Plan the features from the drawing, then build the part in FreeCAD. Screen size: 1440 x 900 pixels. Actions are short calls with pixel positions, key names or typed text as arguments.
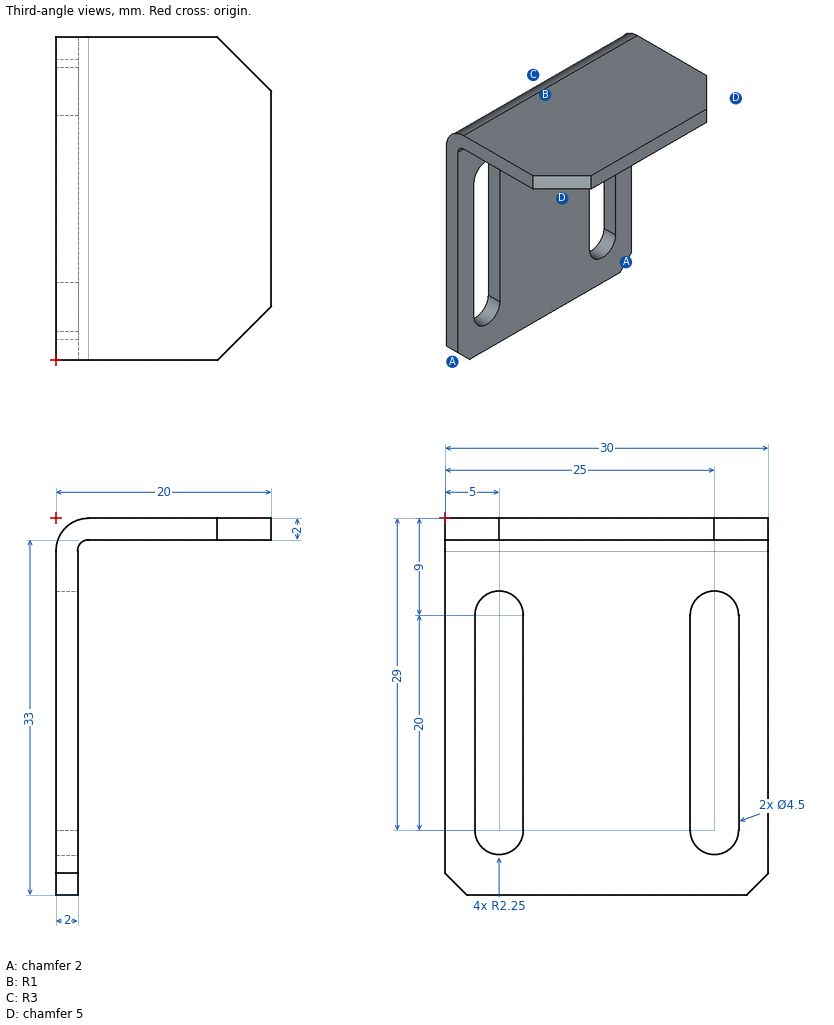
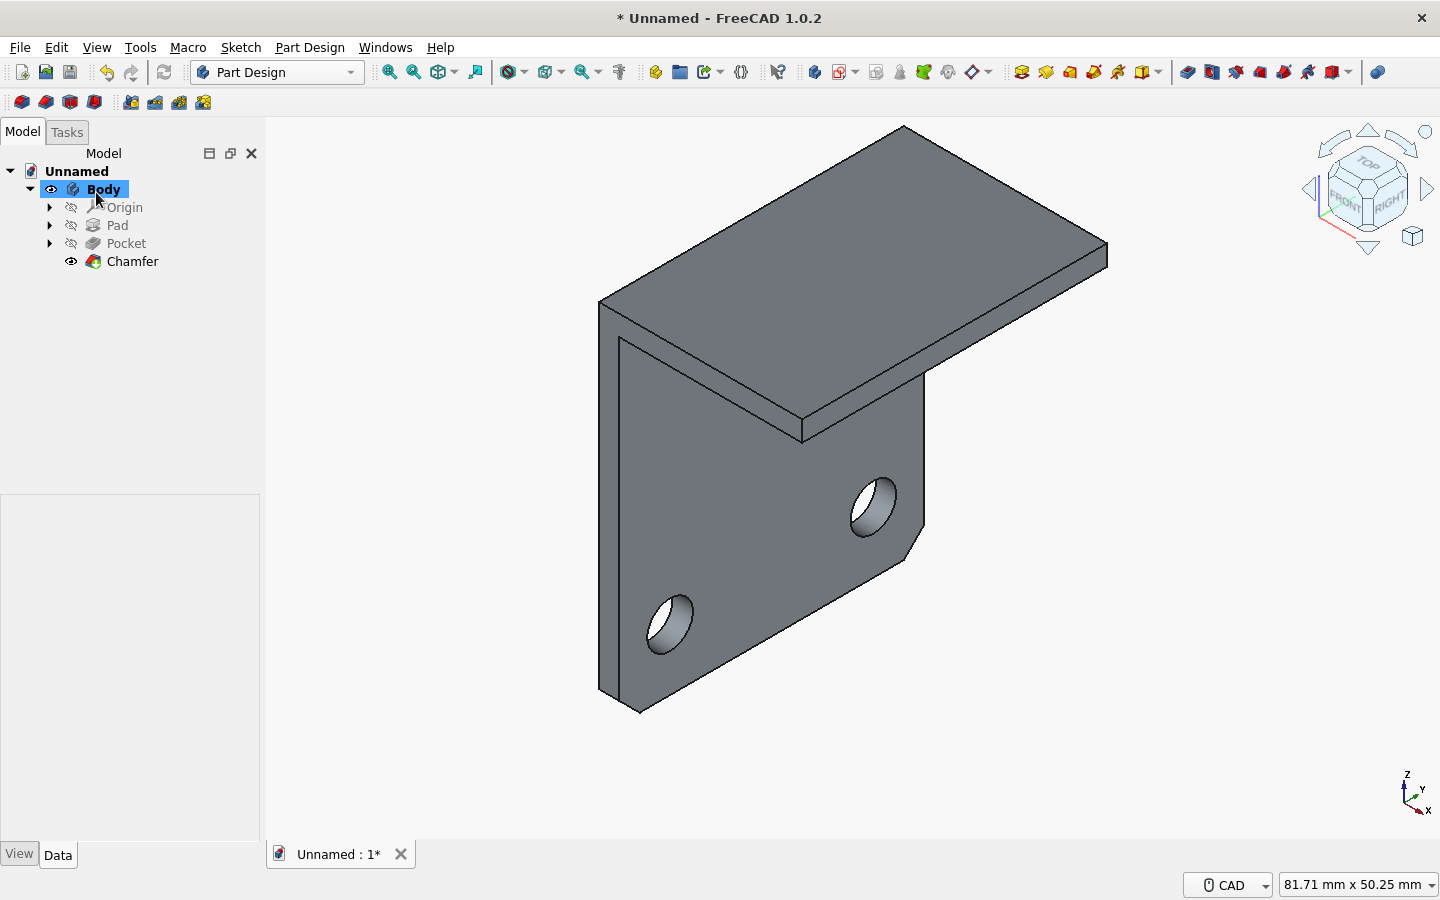
key(2)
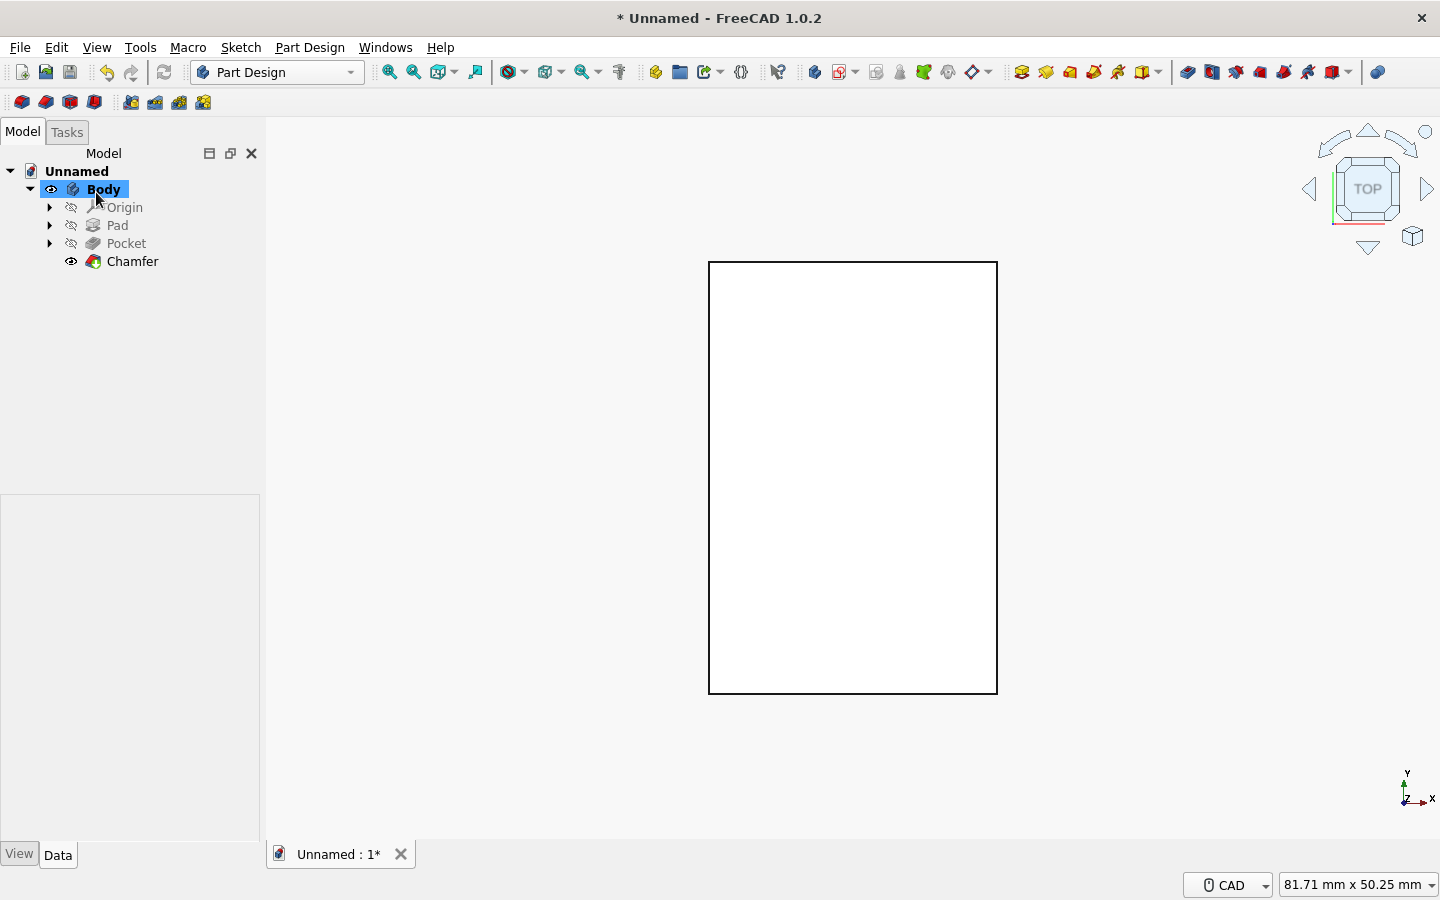
key(1)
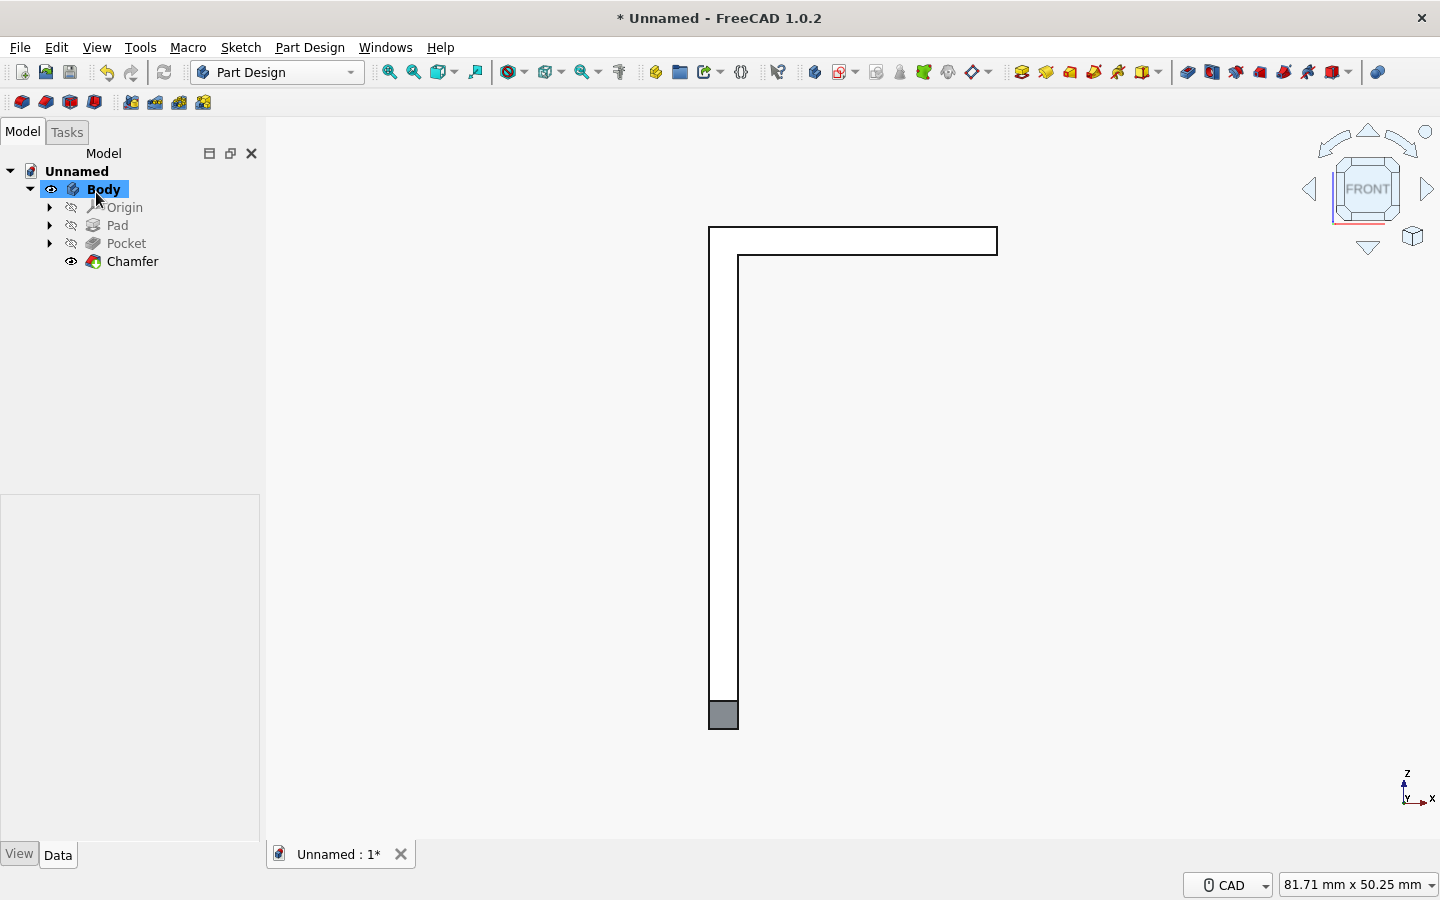
key(3)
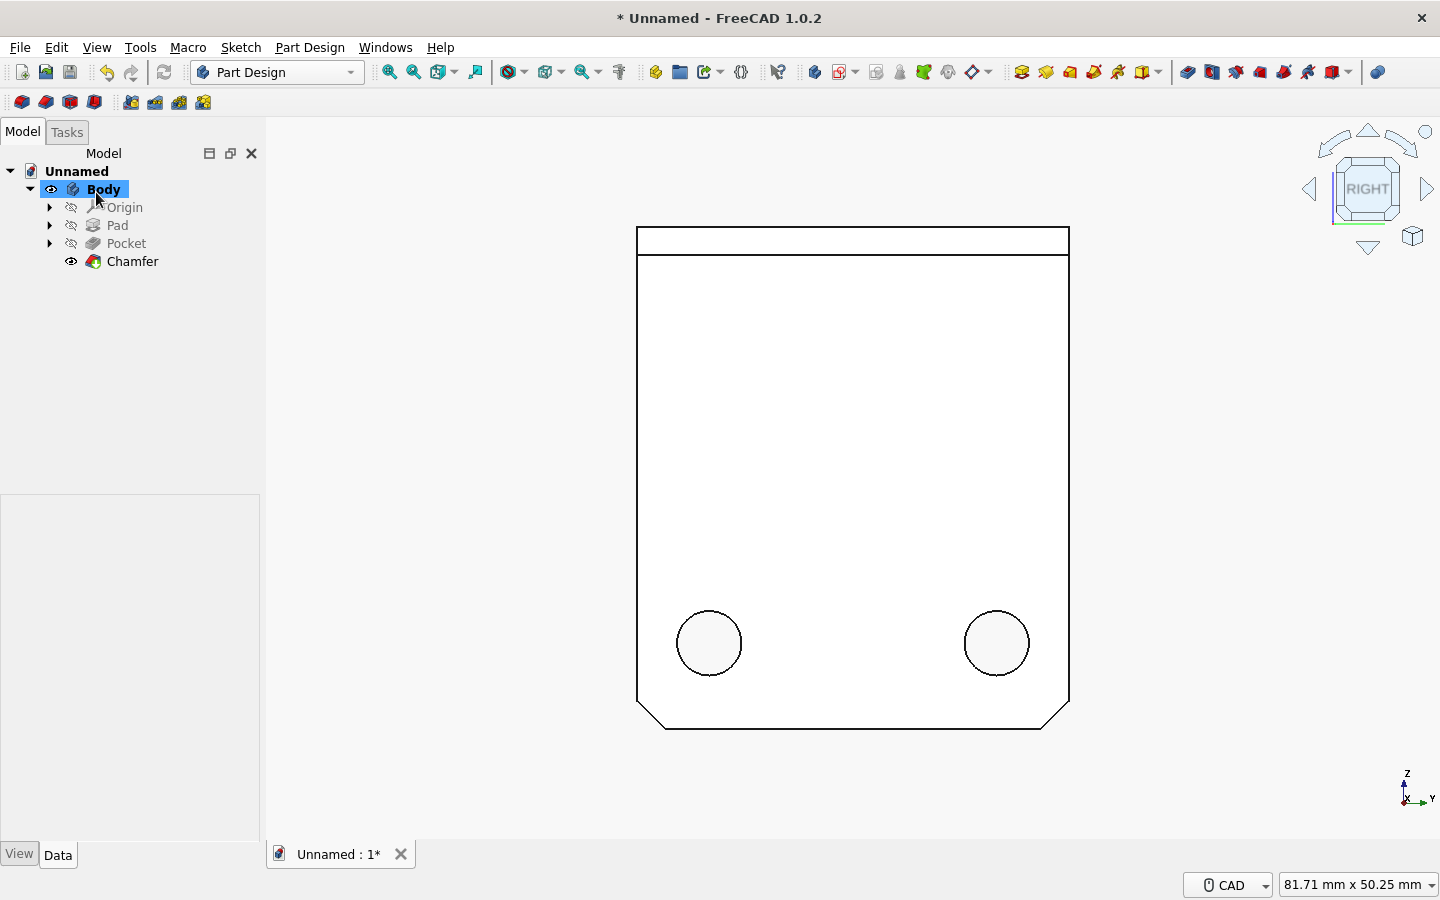
key(5)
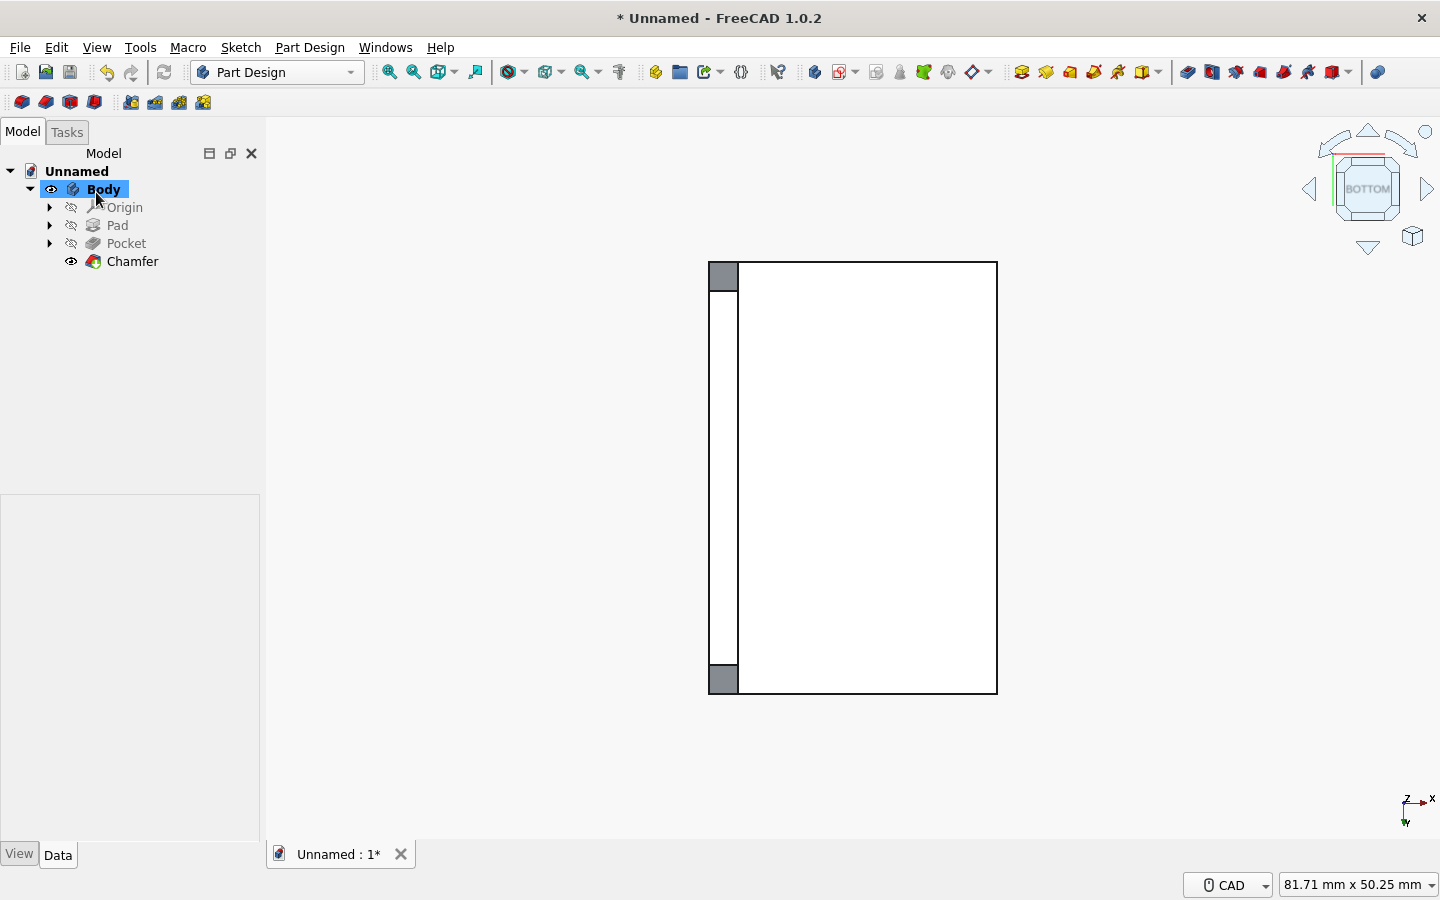
key(4)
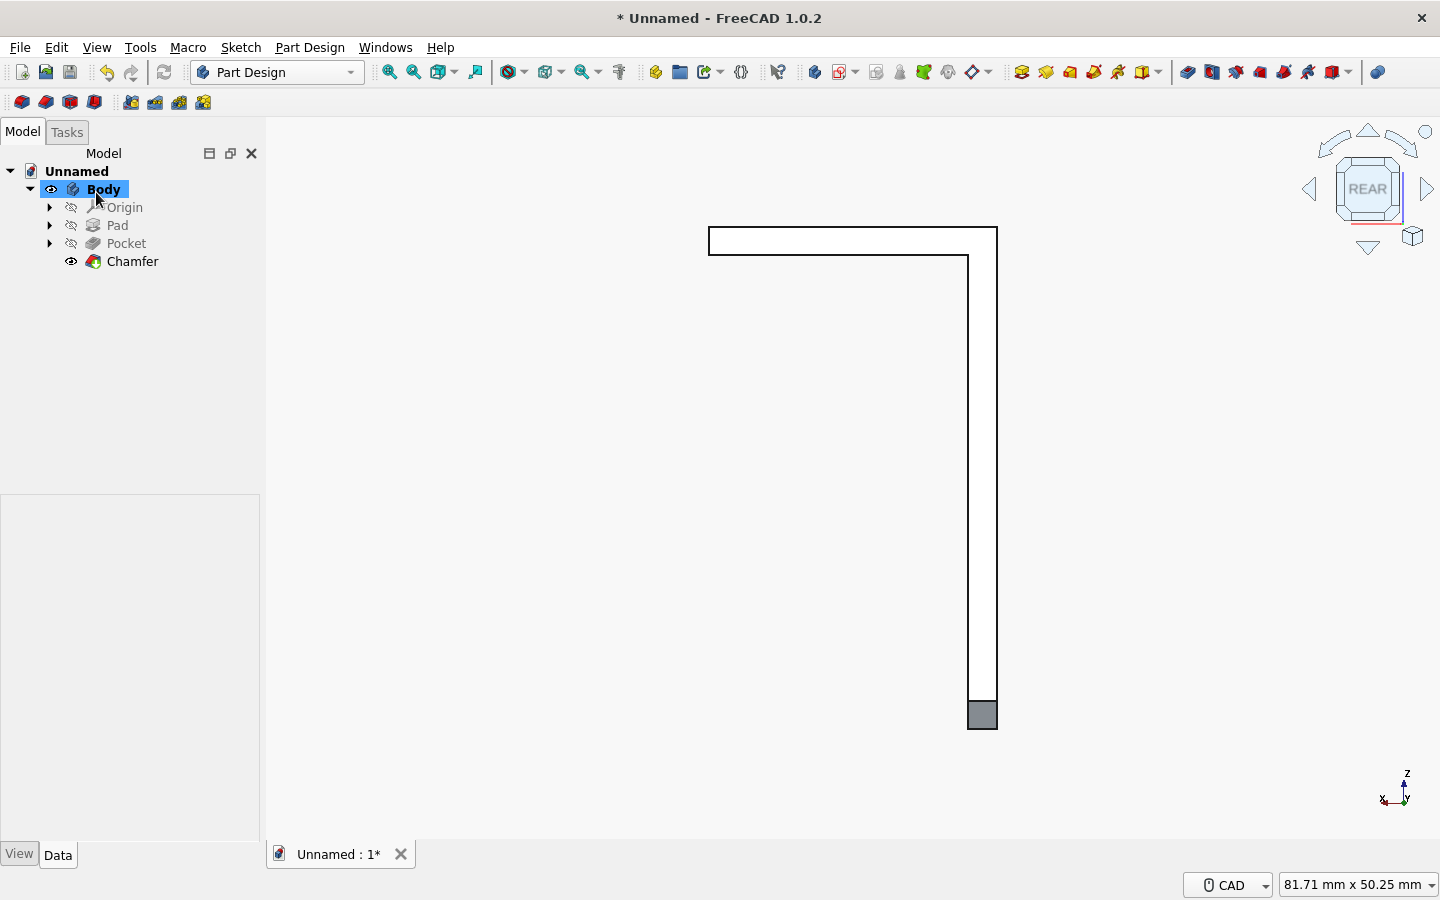
key(6)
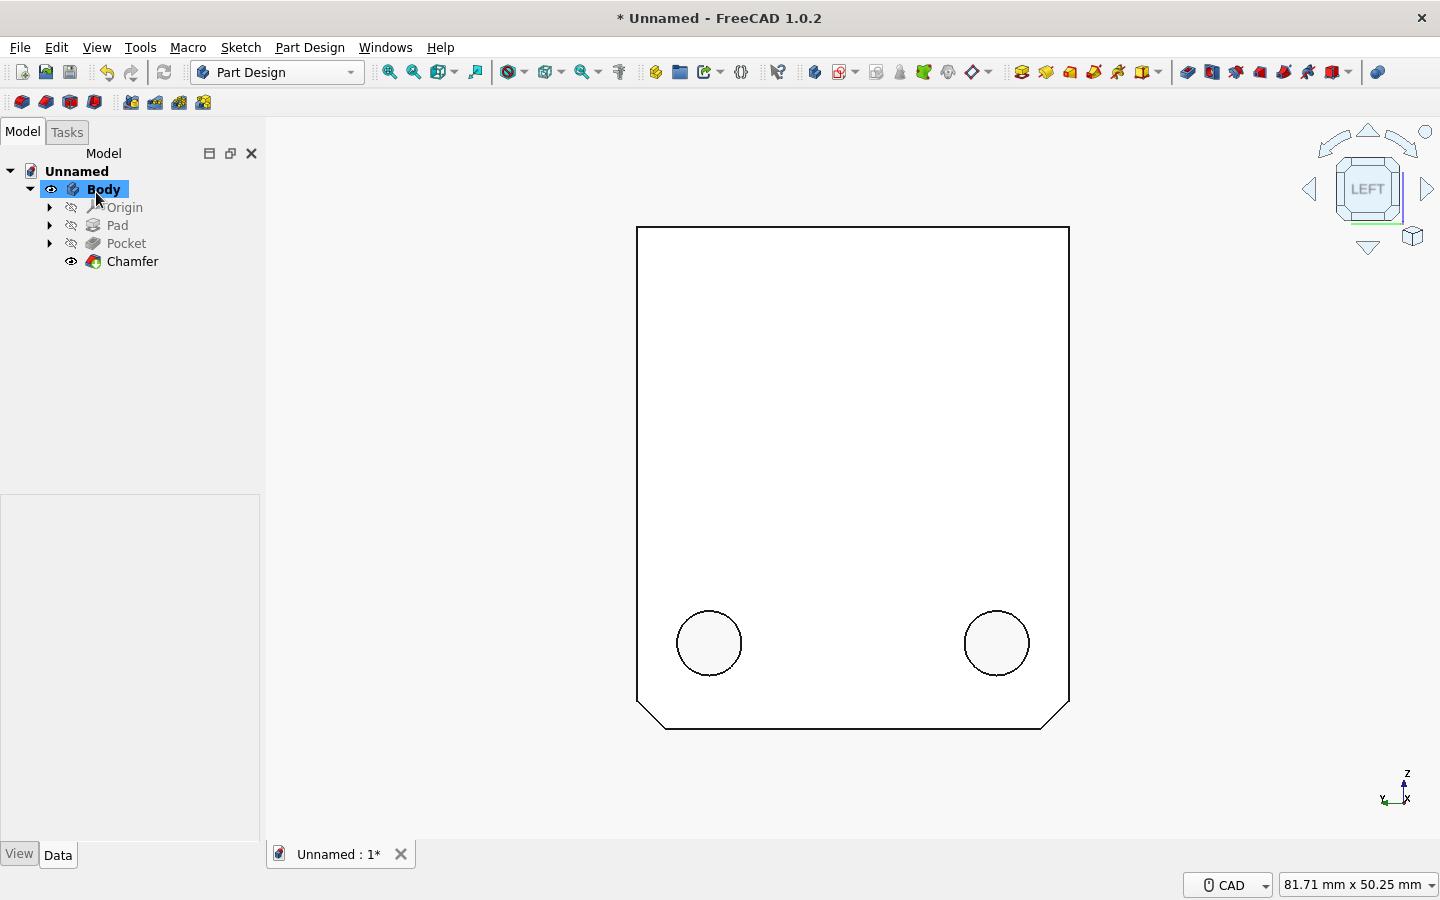
key(v)
key(3)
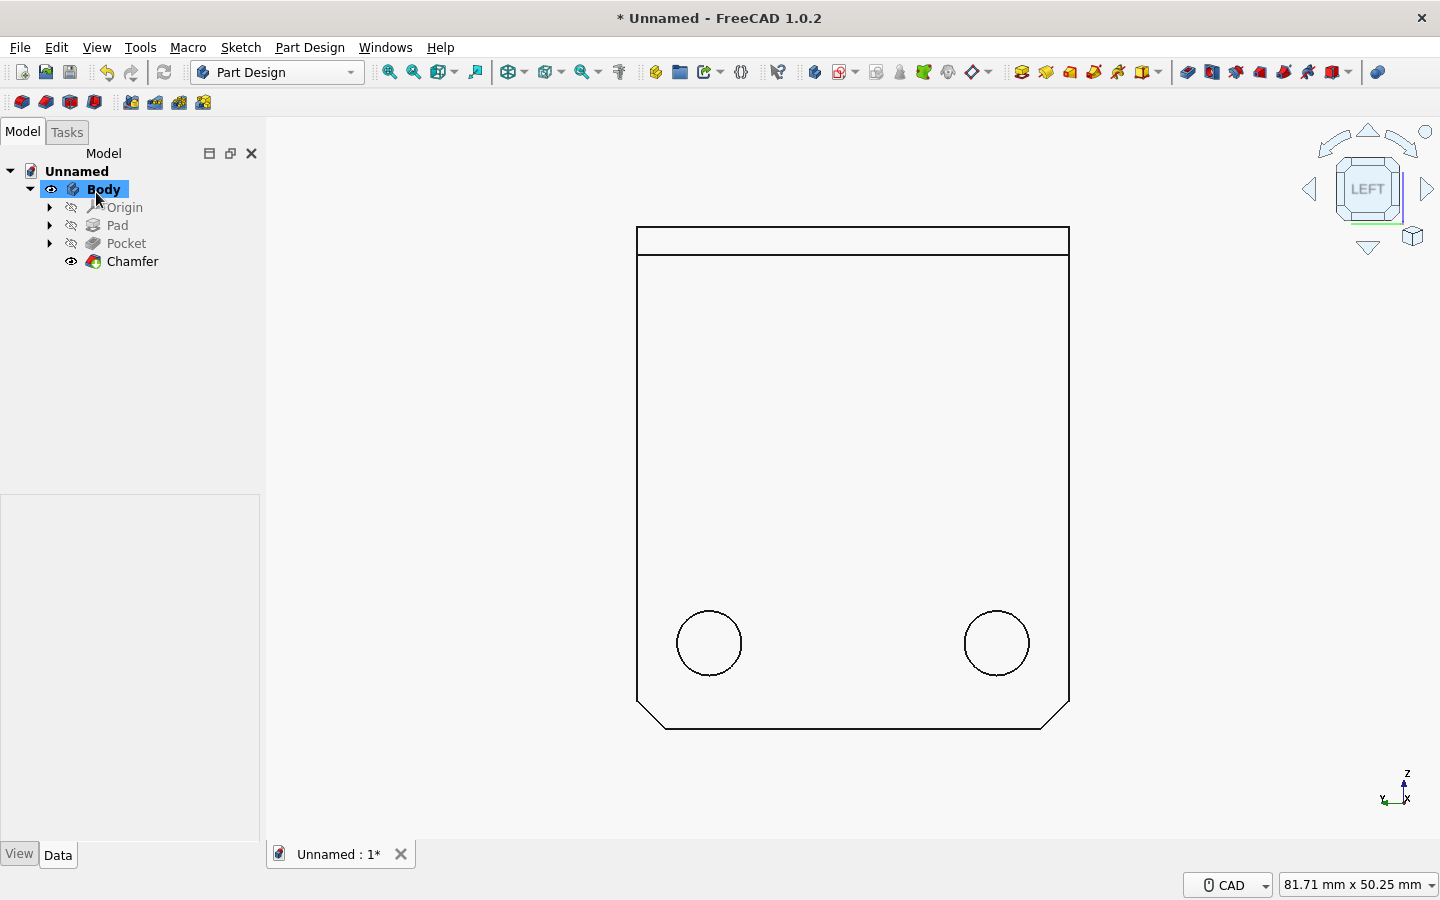
key(0)